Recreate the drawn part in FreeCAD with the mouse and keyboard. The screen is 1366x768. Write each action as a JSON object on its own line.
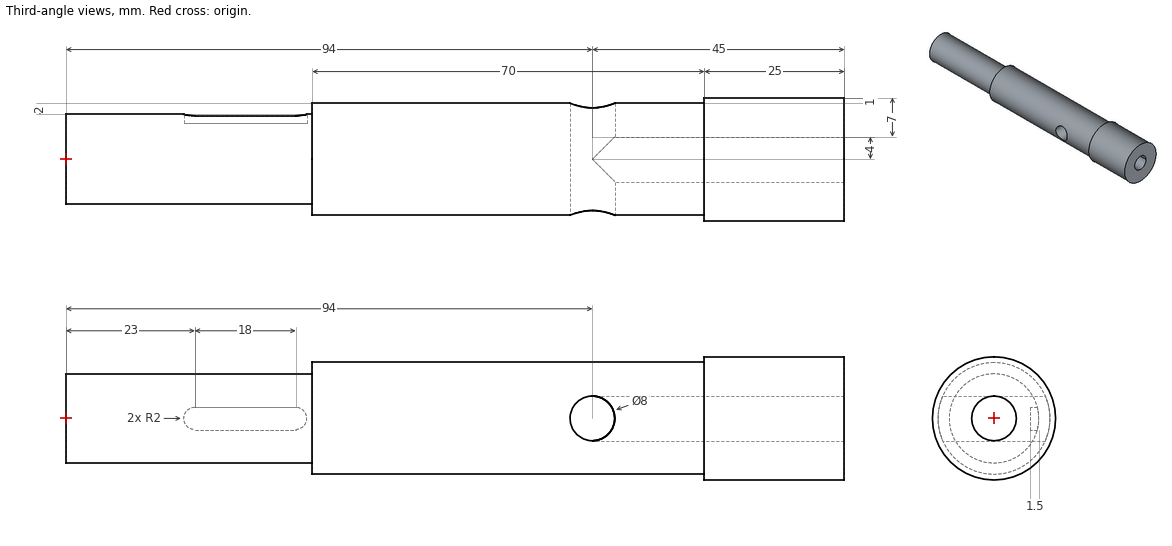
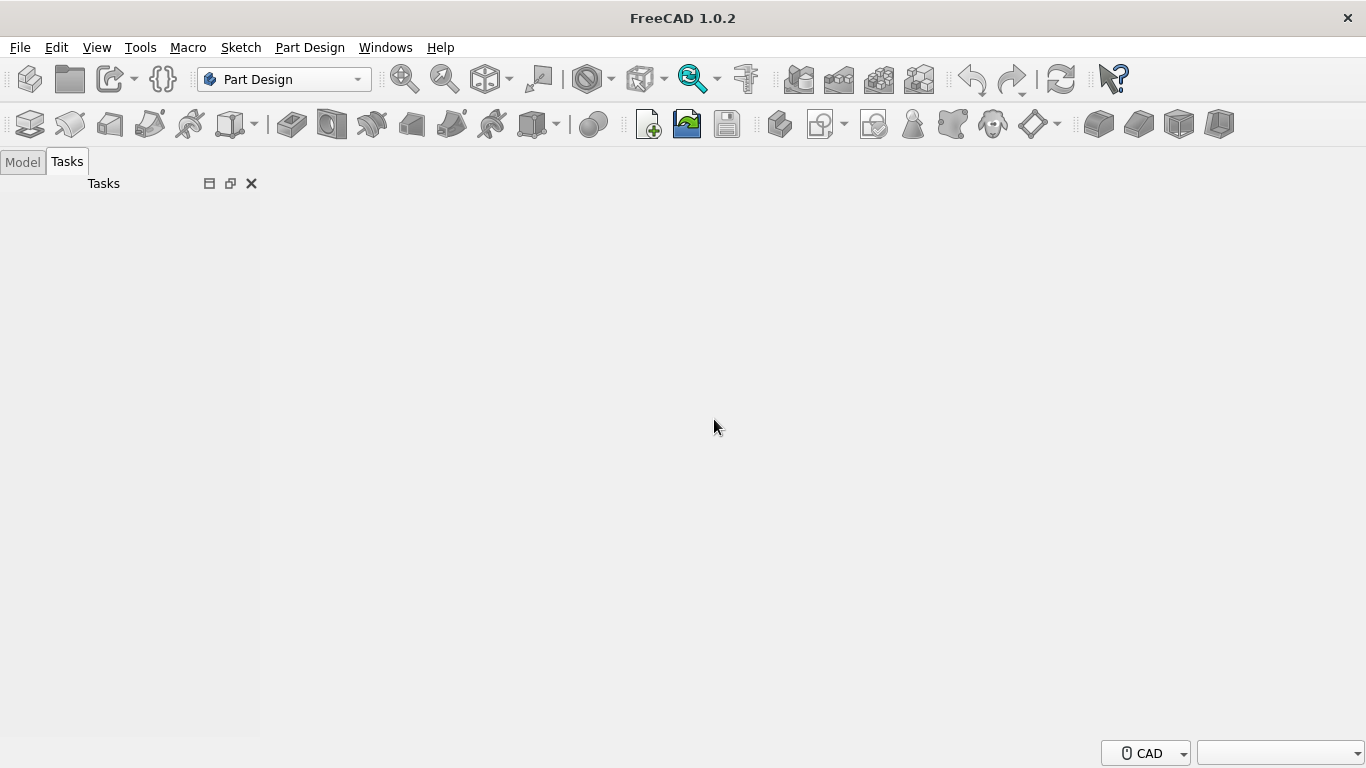
{"action": "key", "text": "ctrl+n"}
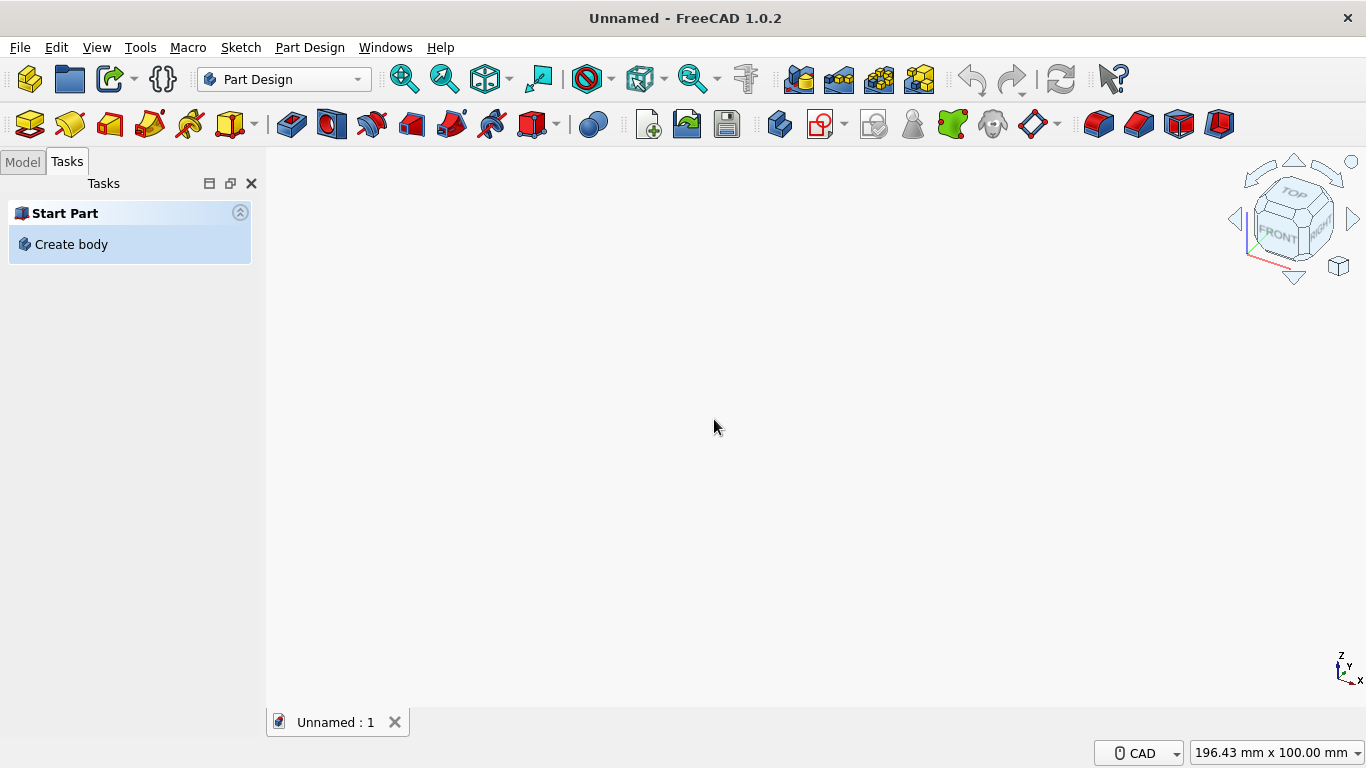
{"action": "left_click", "coordinate": [820, 124]}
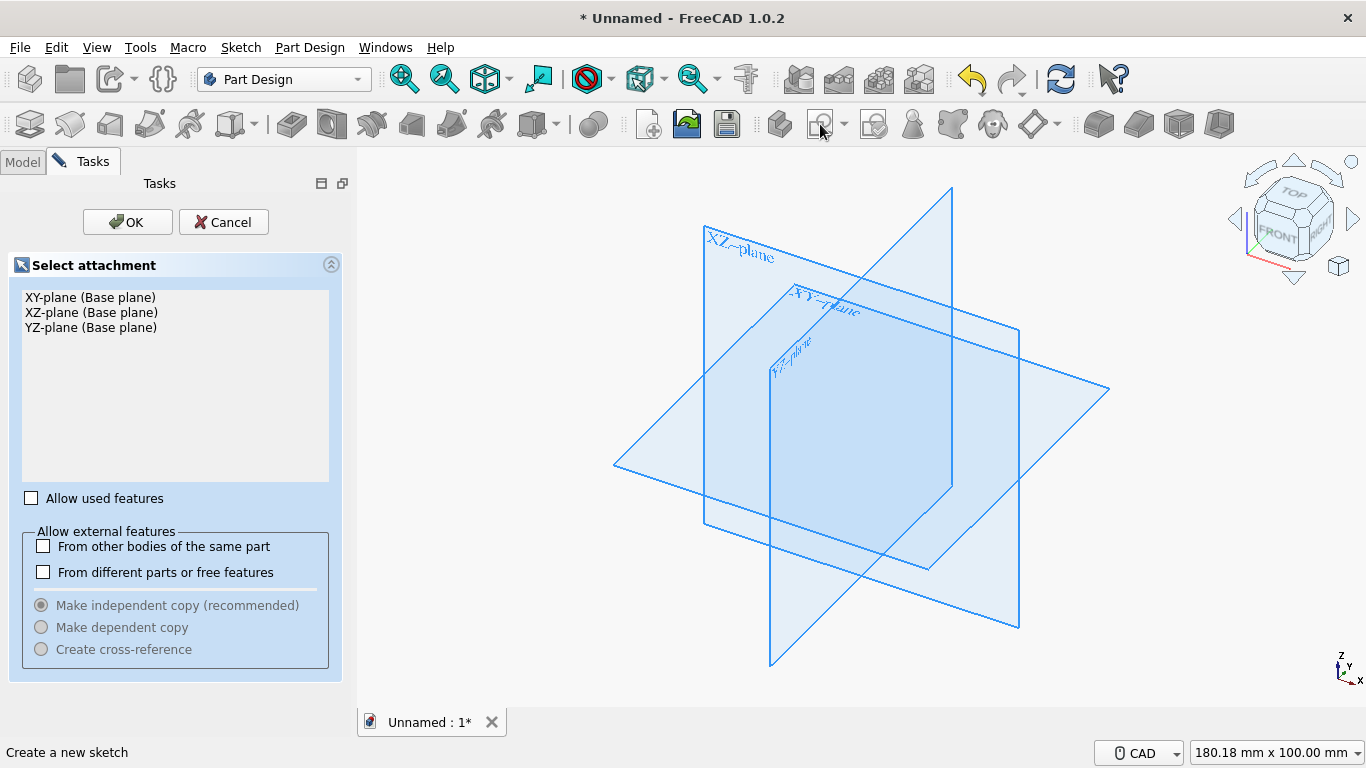
{"action": "left_click", "coordinate": [82, 298]}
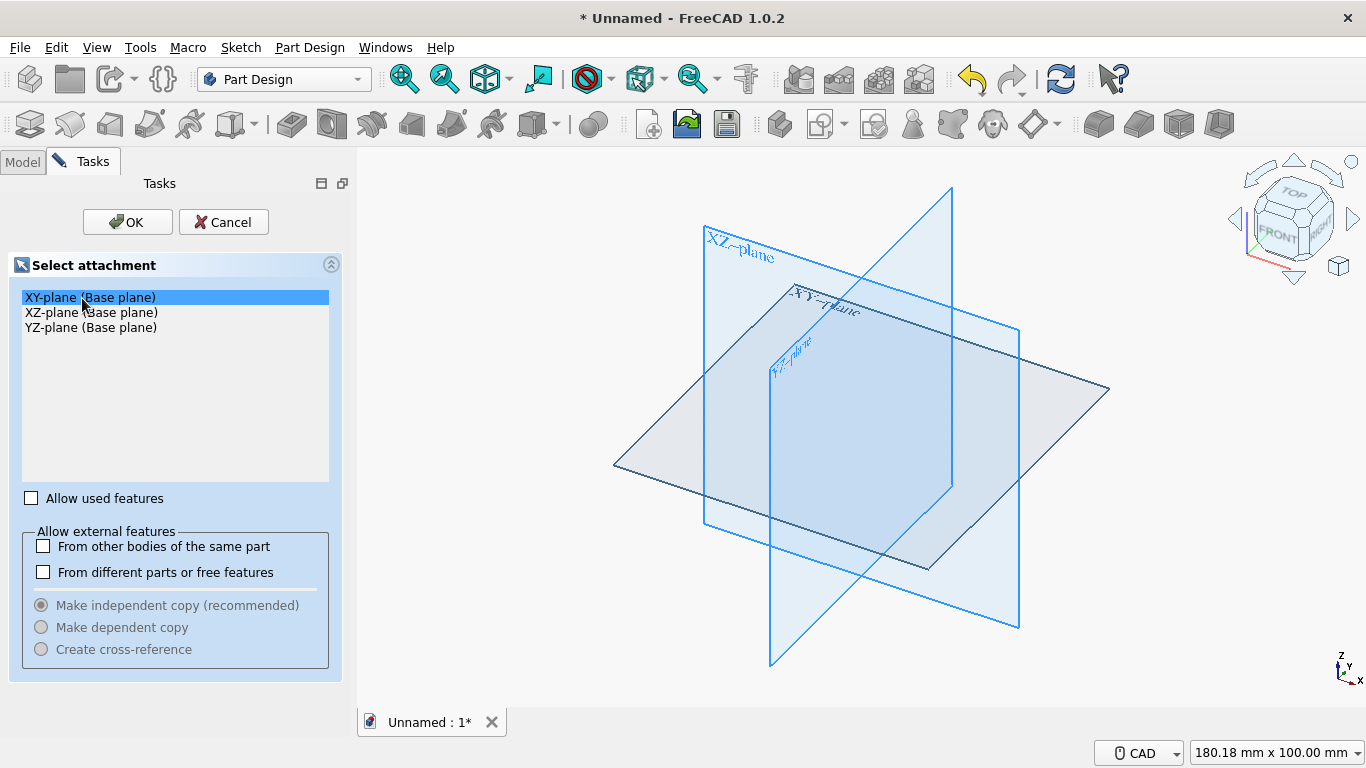
{"action": "left_click", "coordinate": [128, 222]}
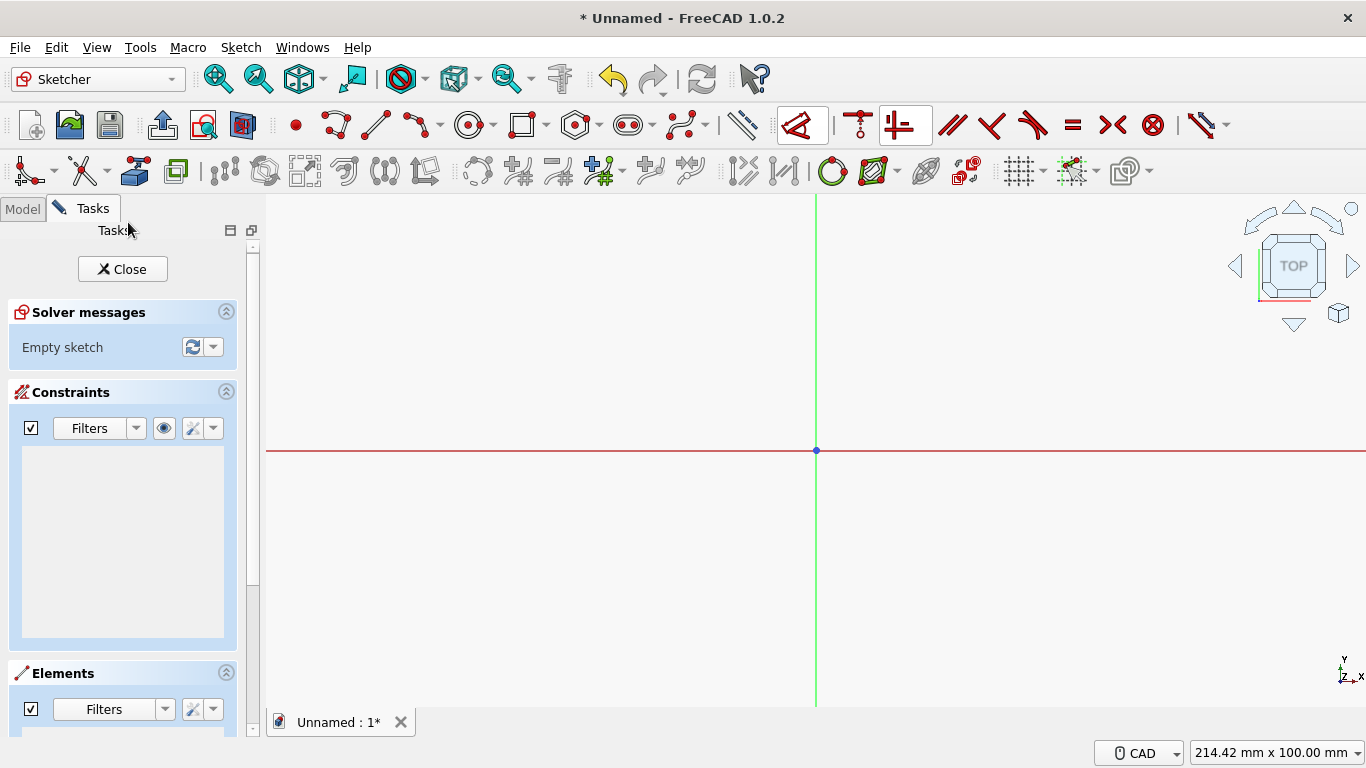
{"action": "scroll", "coordinate": [294, 508], "scroll_direction": "down", "scroll_amount": 2}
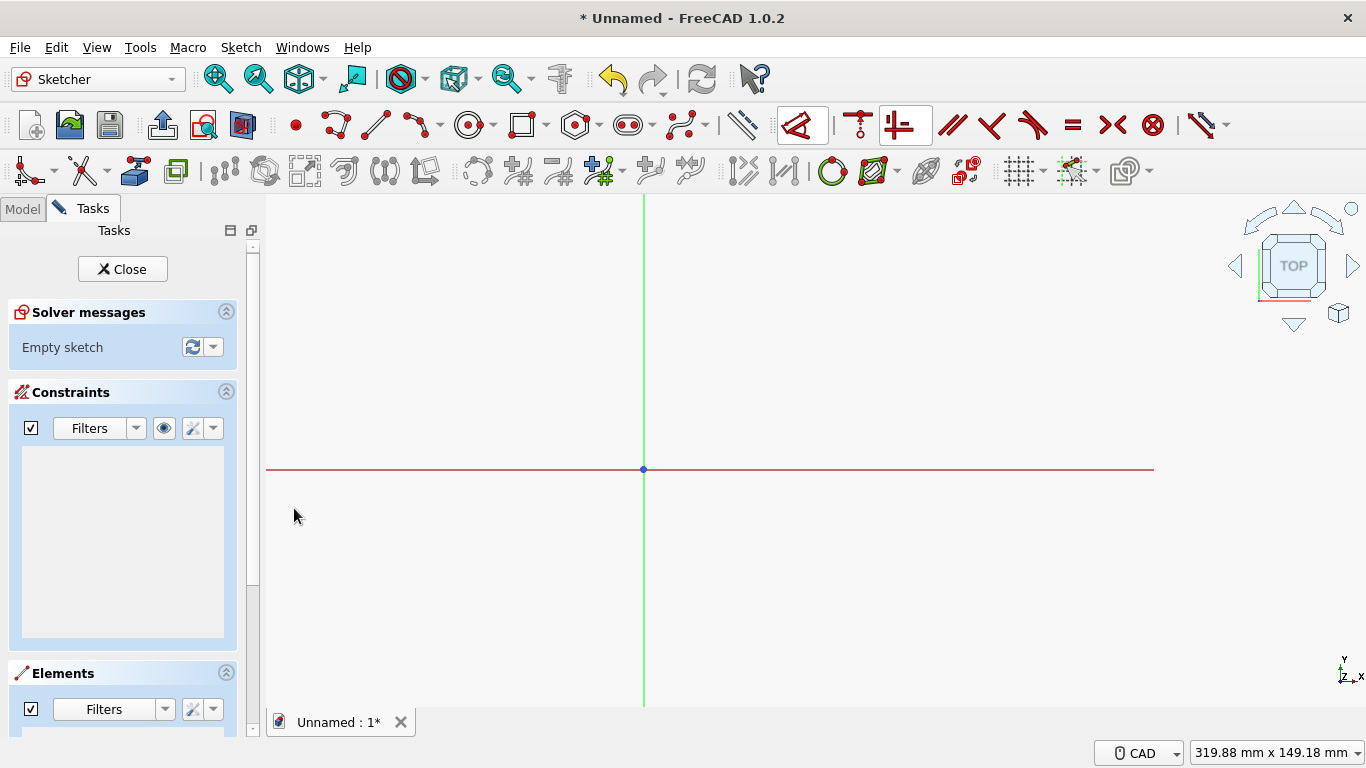
{"action": "left_click", "coordinate": [336, 126]}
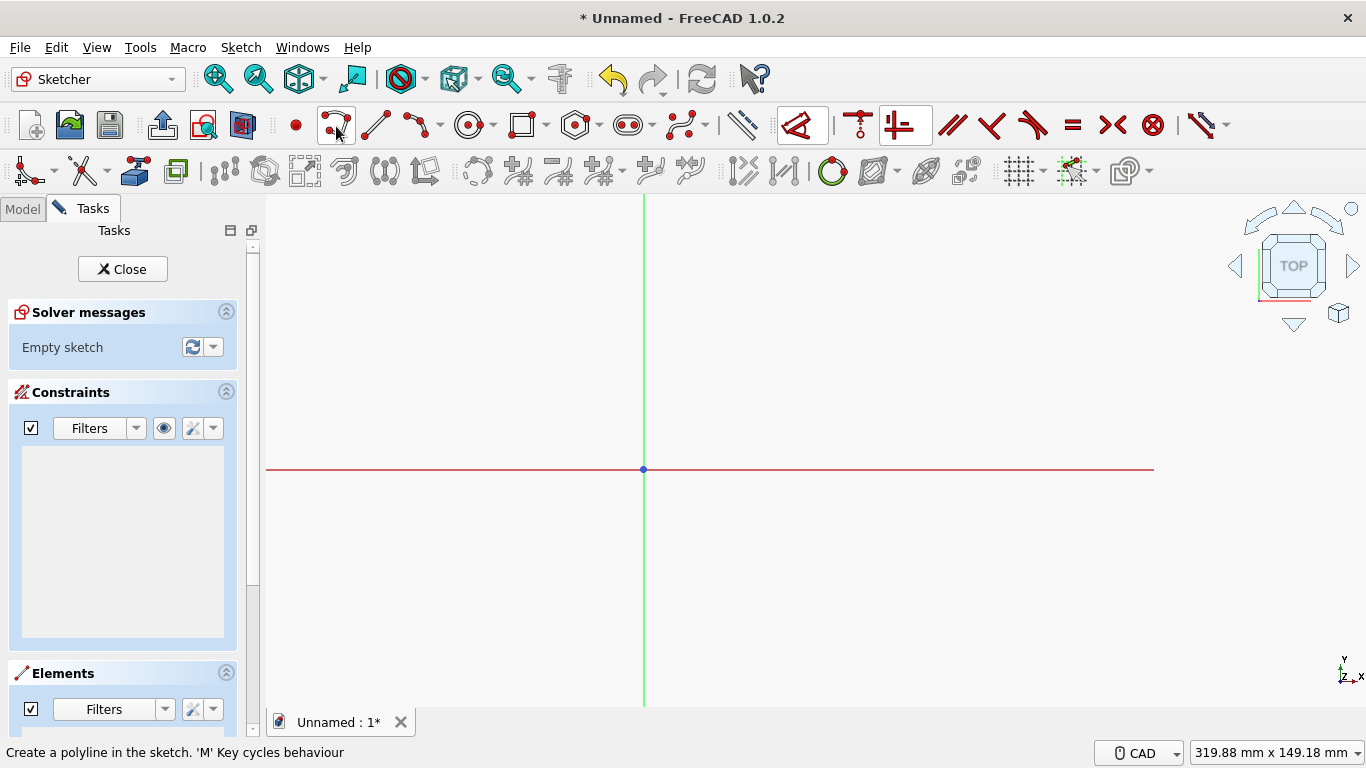
{"action": "left_click", "coordinate": [644, 470]}
{"action": "left_click", "coordinate": [967, 461]}
{"action": "left_click", "coordinate": [967, 456]}
{"action": "left_click", "coordinate": [1122, 456]}
{"action": "left_click", "coordinate": [1122, 432]}
{"action": "left_click", "coordinate": [1036, 432]}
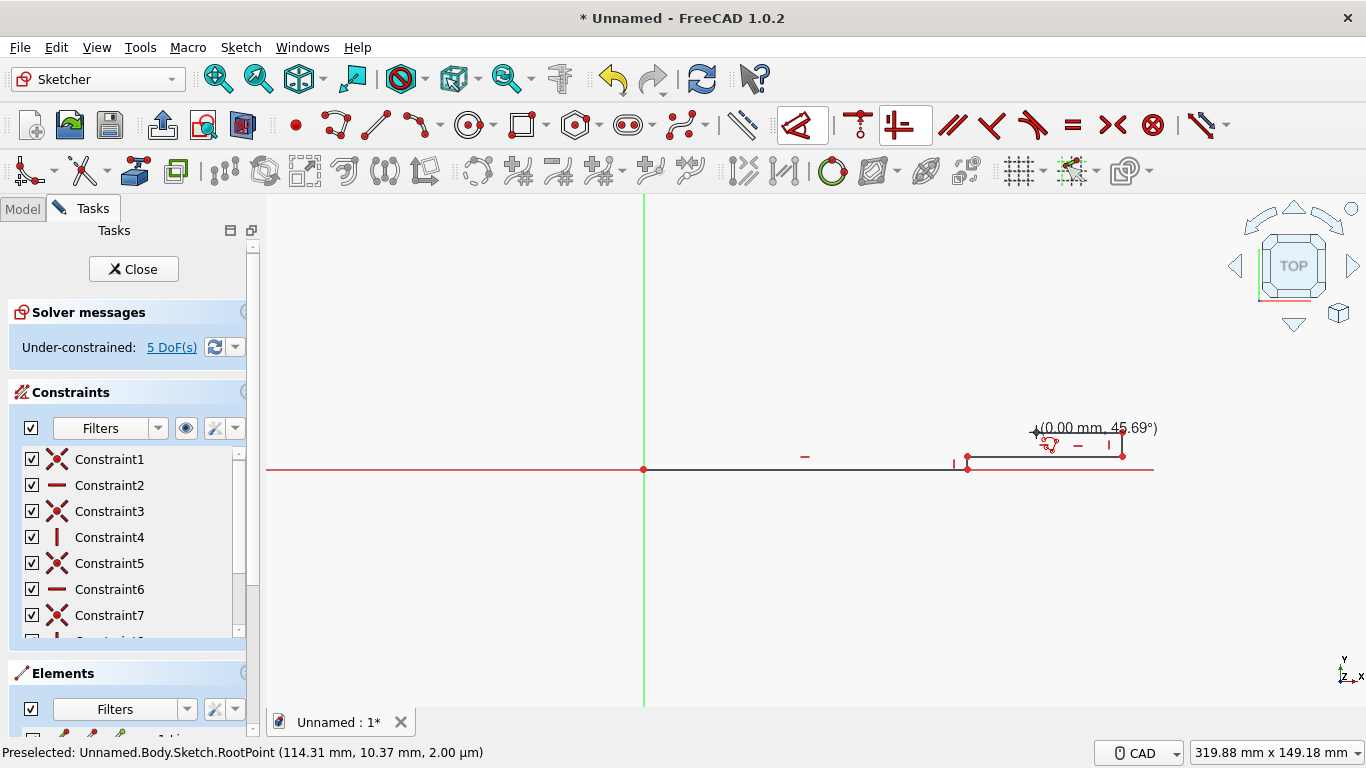
{"action": "scroll", "coordinate": [1036, 435], "scroll_direction": "up", "scroll_amount": 8}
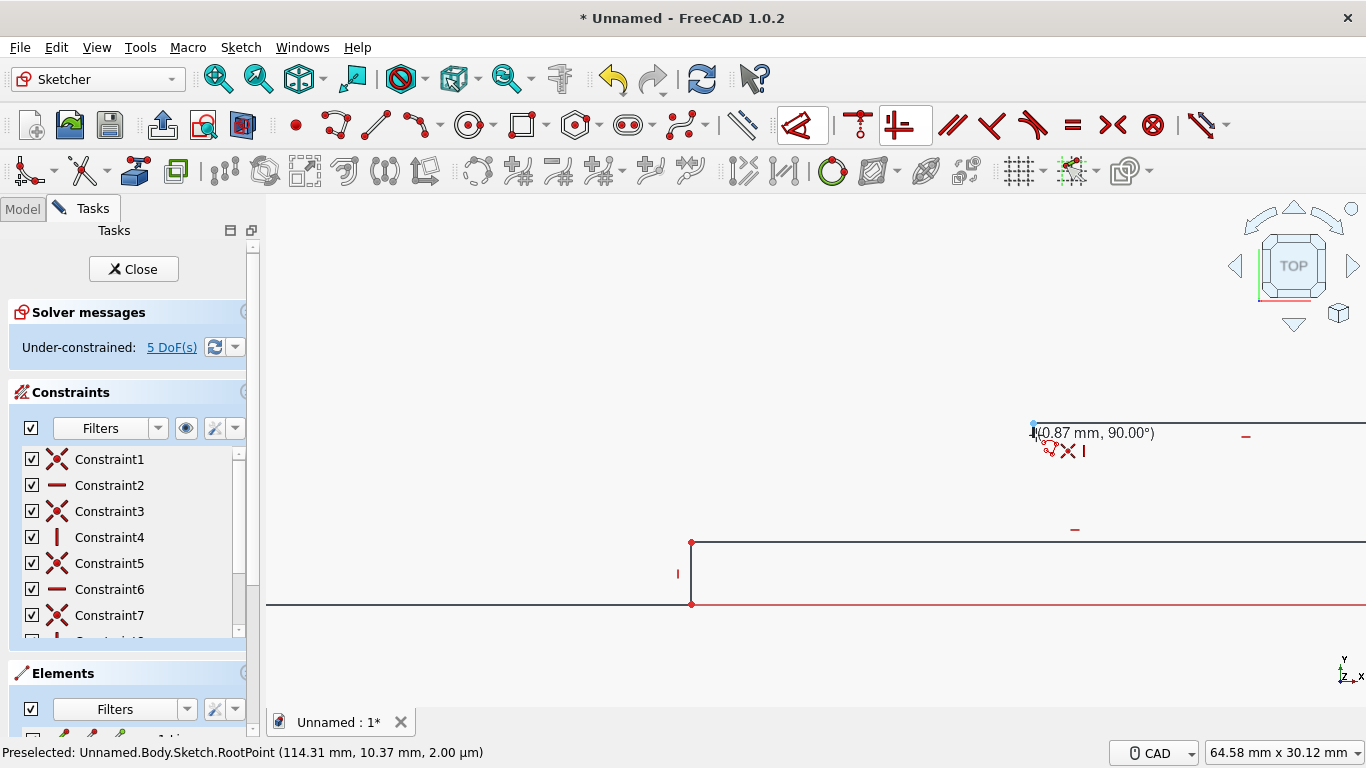
{"action": "left_click", "coordinate": [1033, 434]}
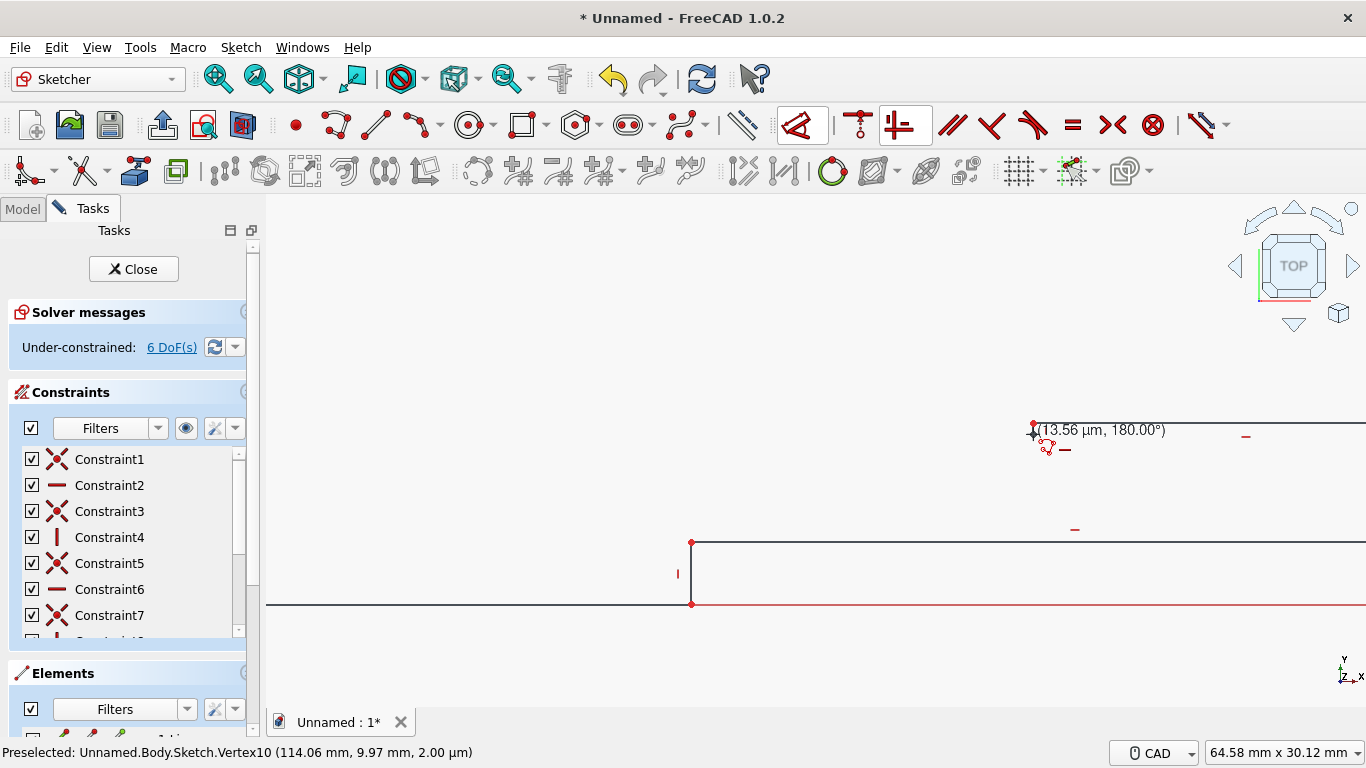
{"action": "scroll", "coordinate": [902, 431], "scroll_direction": "down", "scroll_amount": 7}